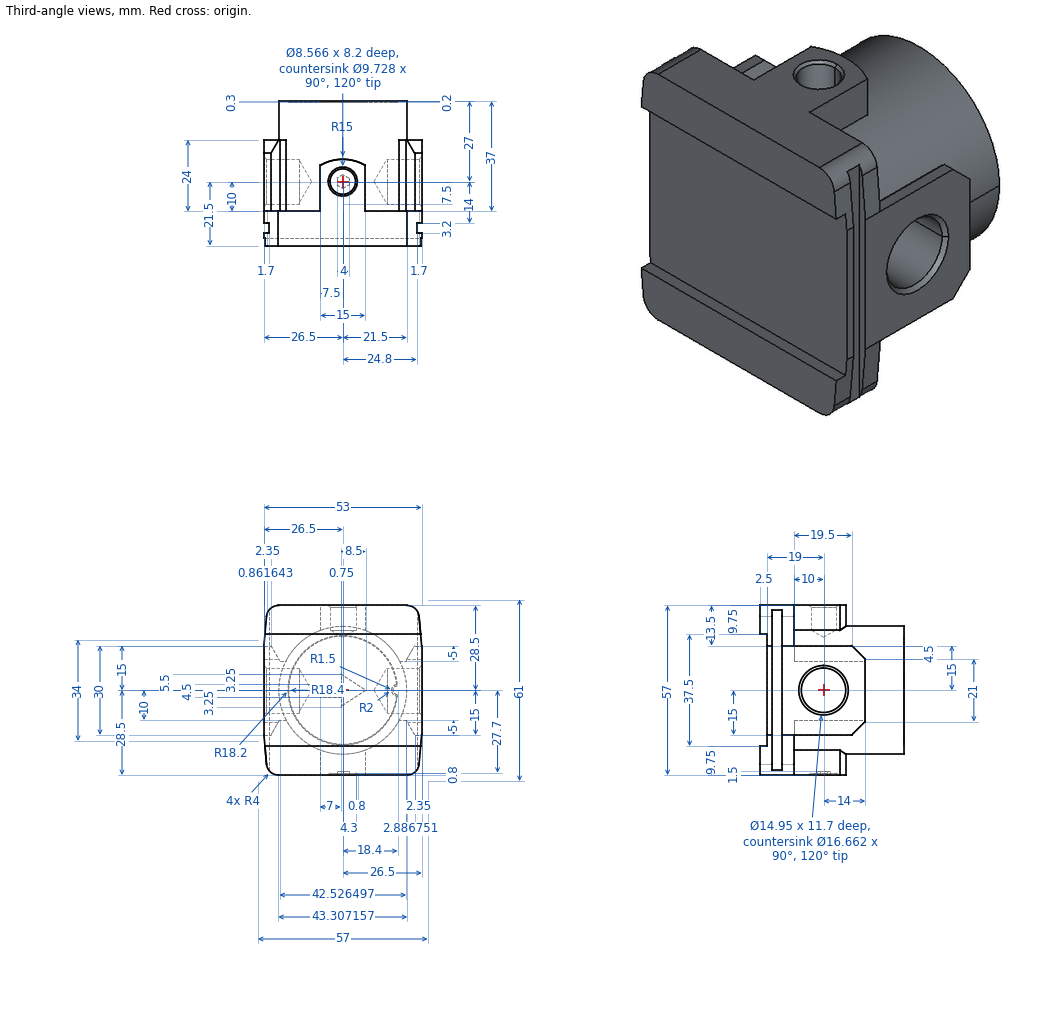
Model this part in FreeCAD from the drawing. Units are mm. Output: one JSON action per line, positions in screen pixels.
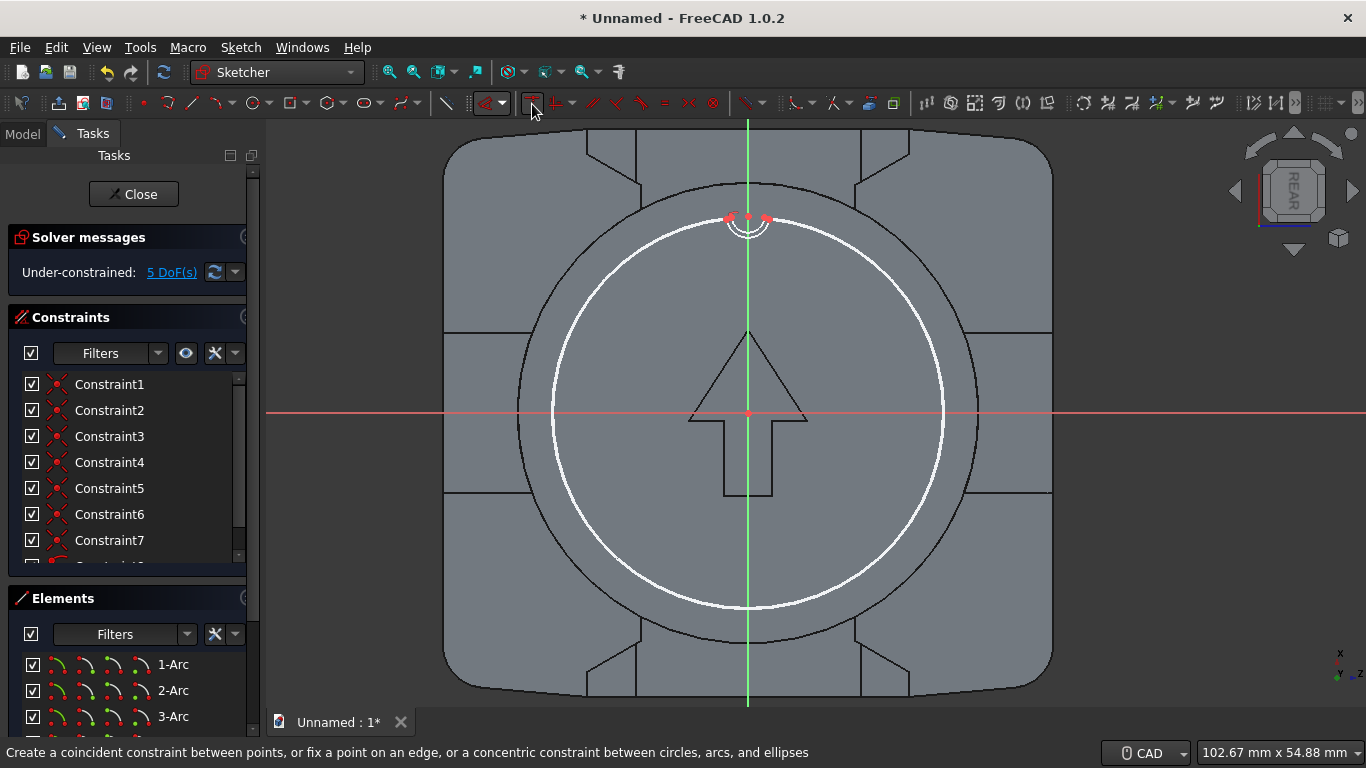
{"action": "scroll", "coordinate": [563, 480], "scroll_direction": "up", "scroll_amount": 12}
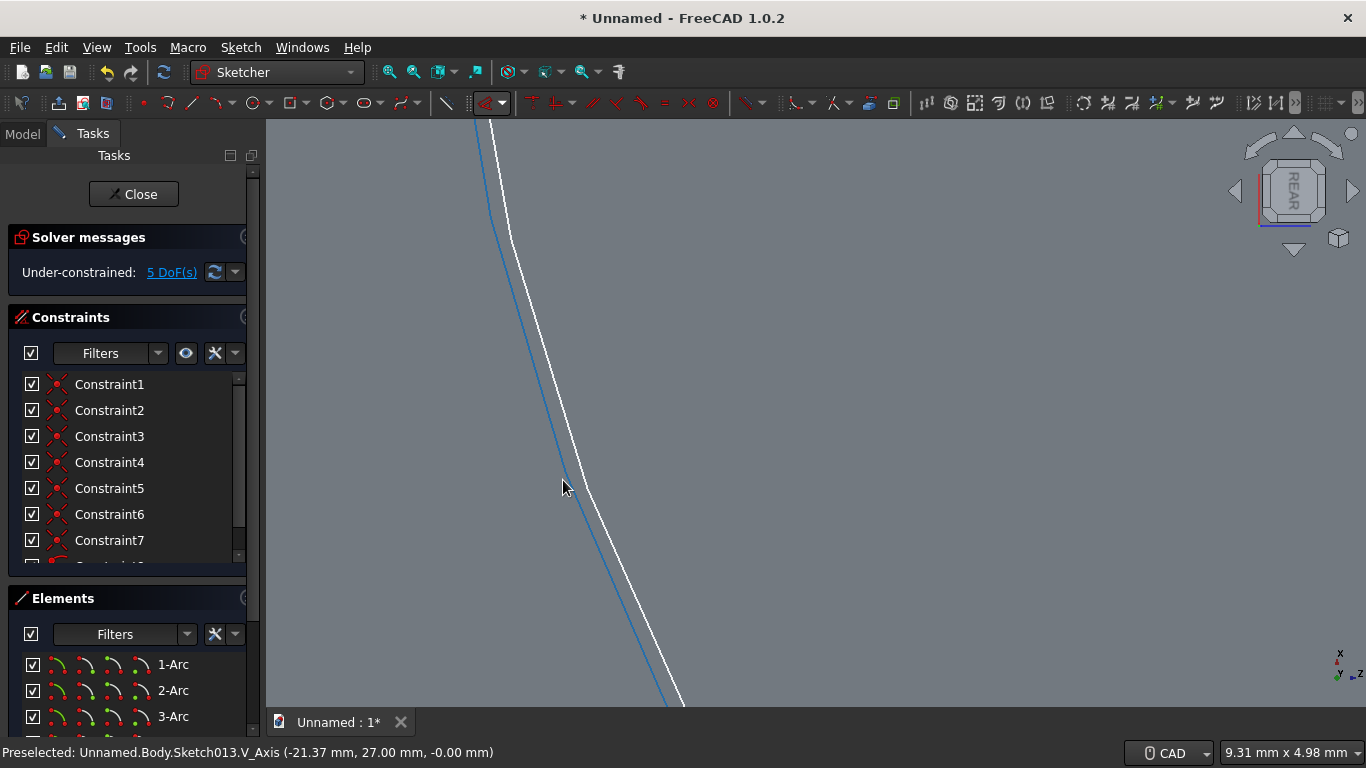
{"action": "left_click", "coordinate": [566, 473]}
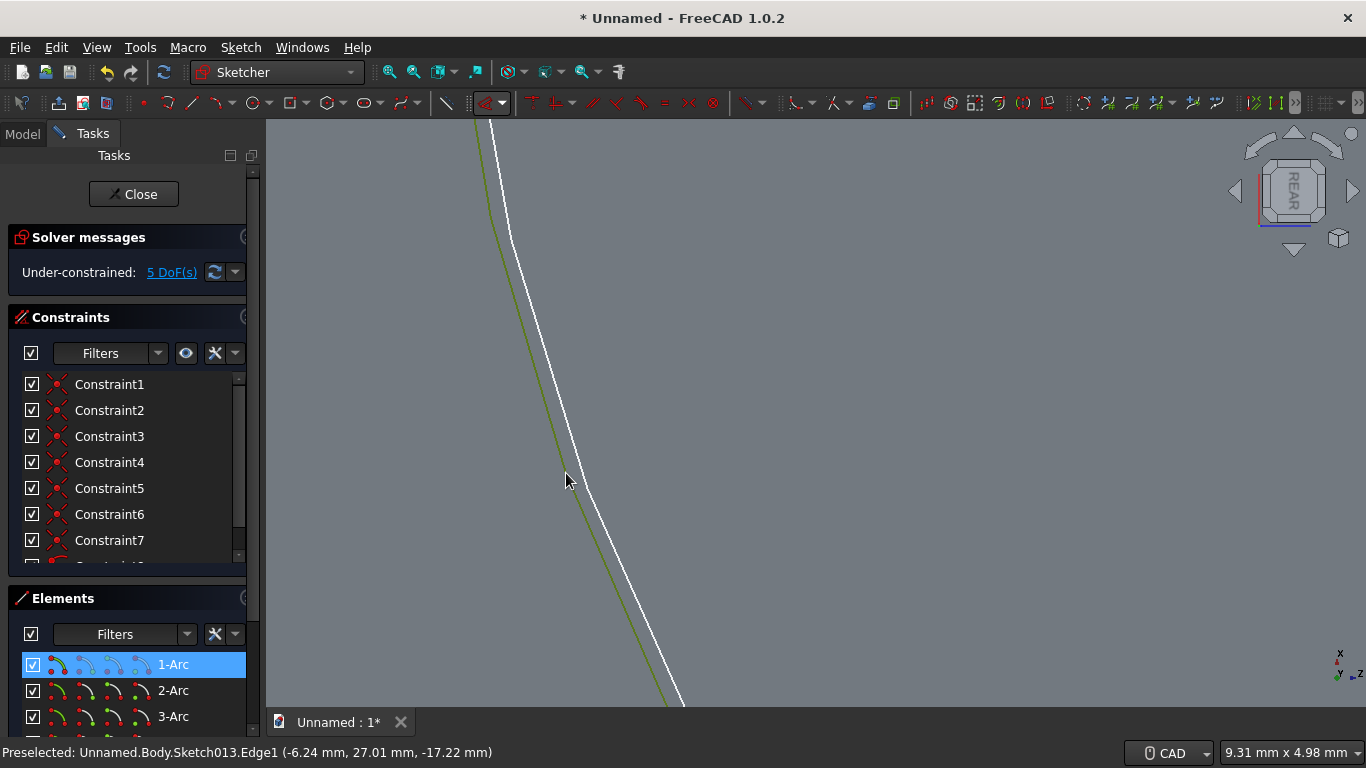
{"action": "left_click", "coordinate": [504, 104]}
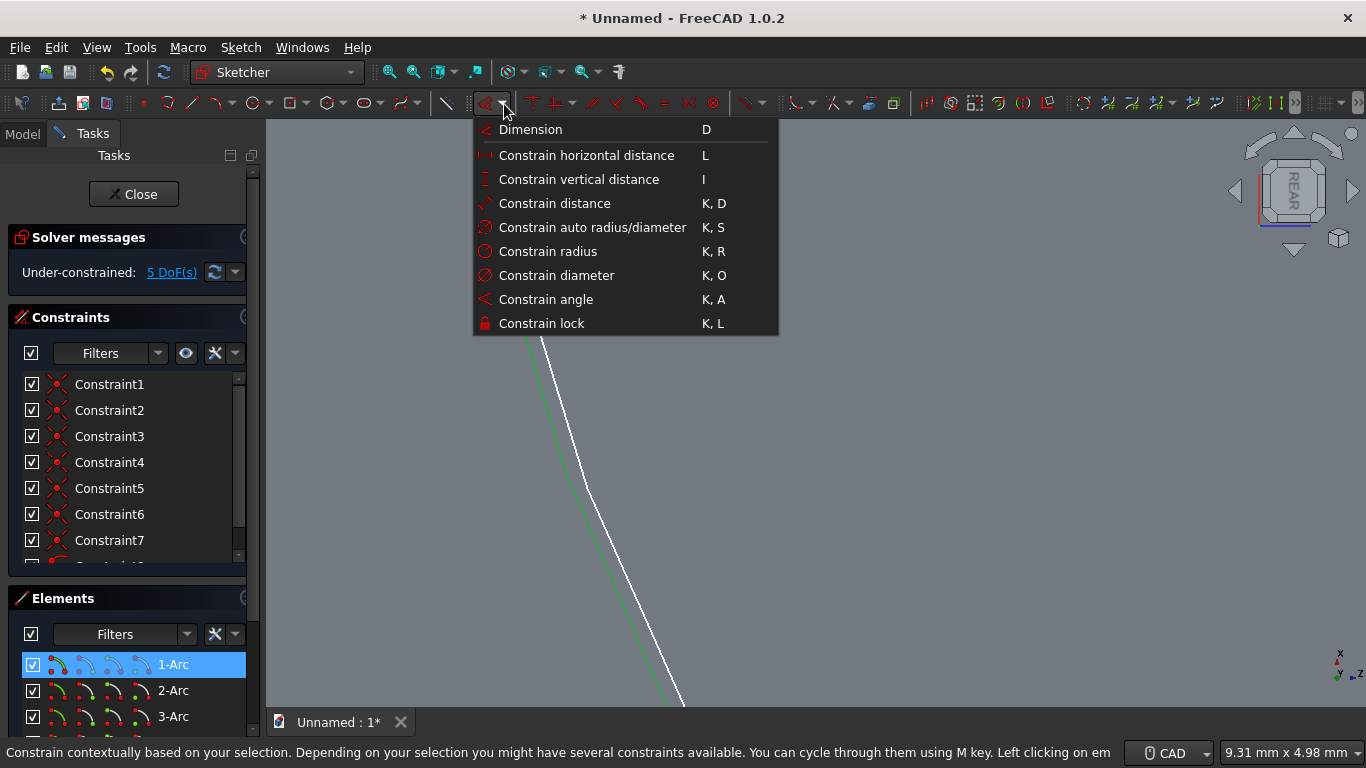
{"action": "left_click", "coordinate": [626, 251]}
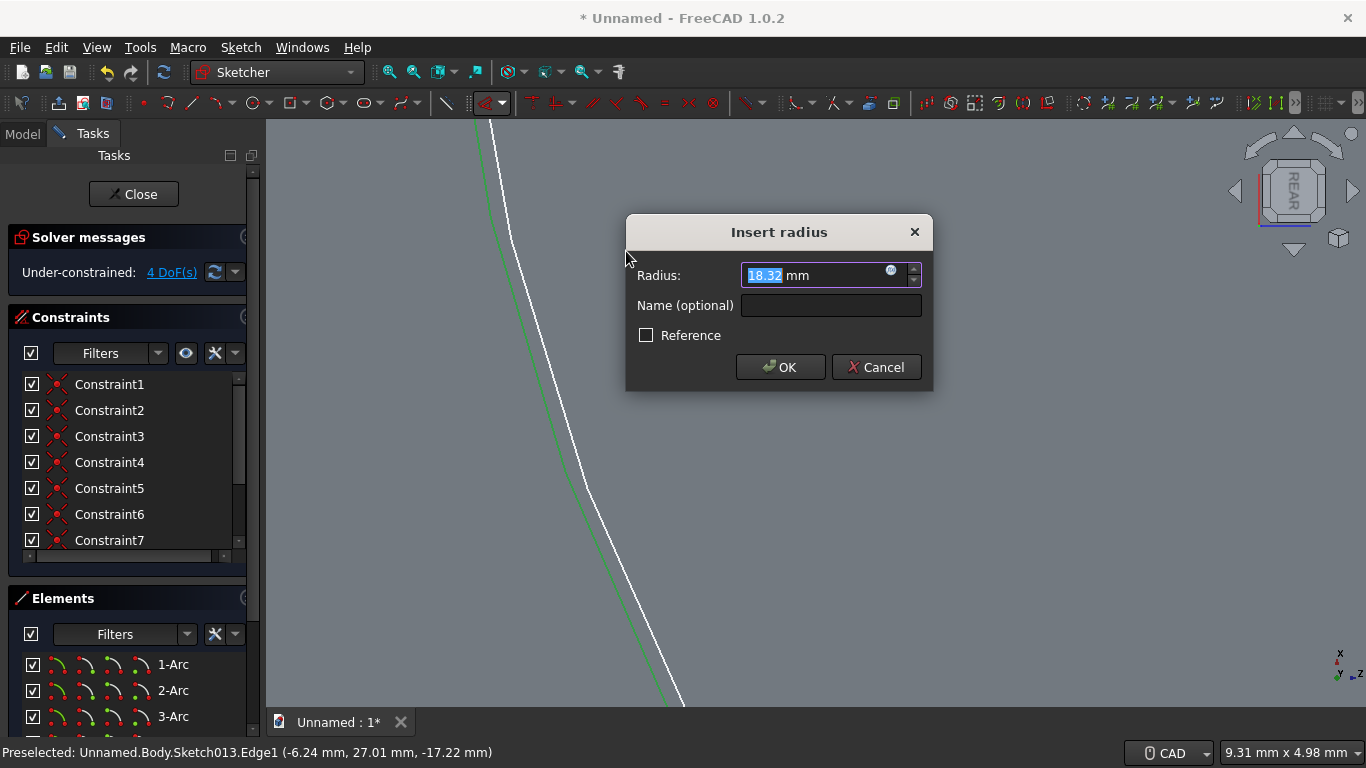
{"action": "type", "text": "18.4"}
{"action": "key", "text": "Return"}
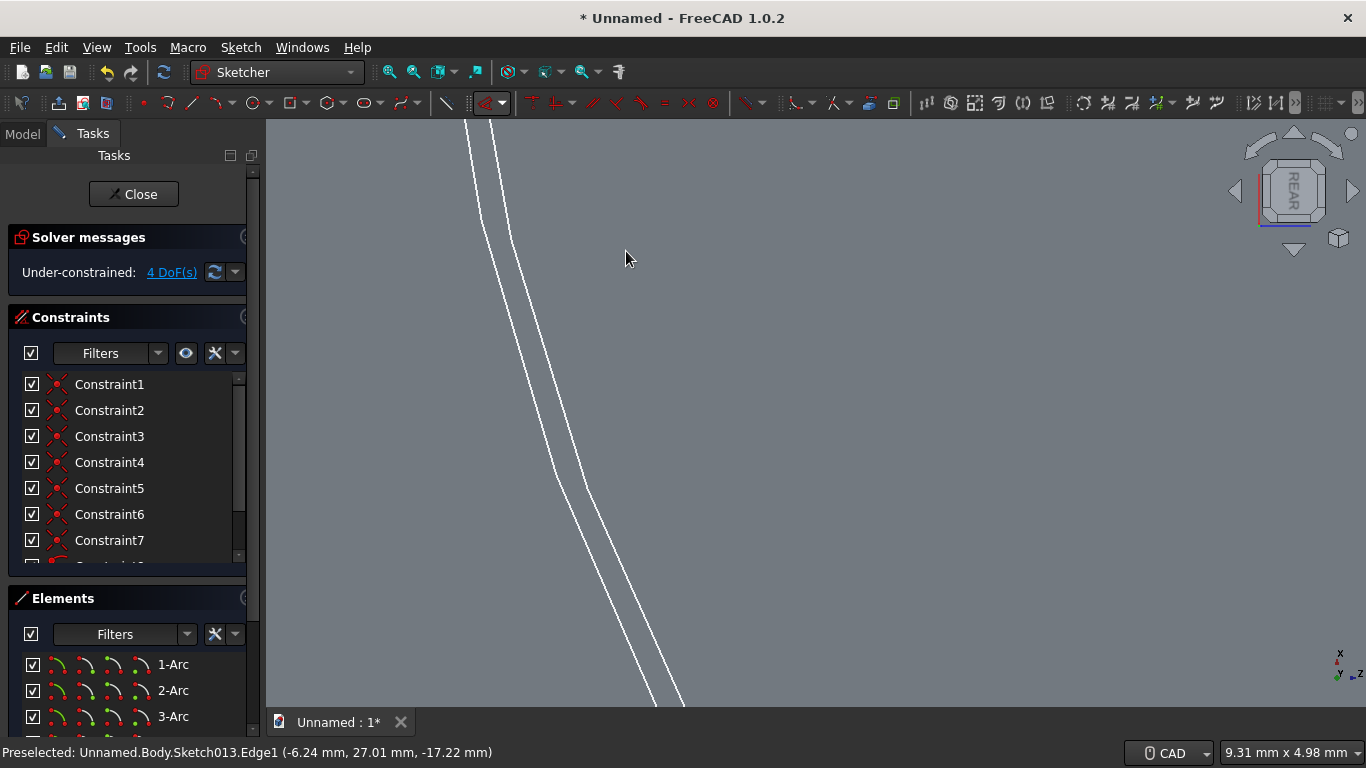
{"action": "scroll", "coordinate": [563, 480], "scroll_direction": "down", "scroll_amount": 12}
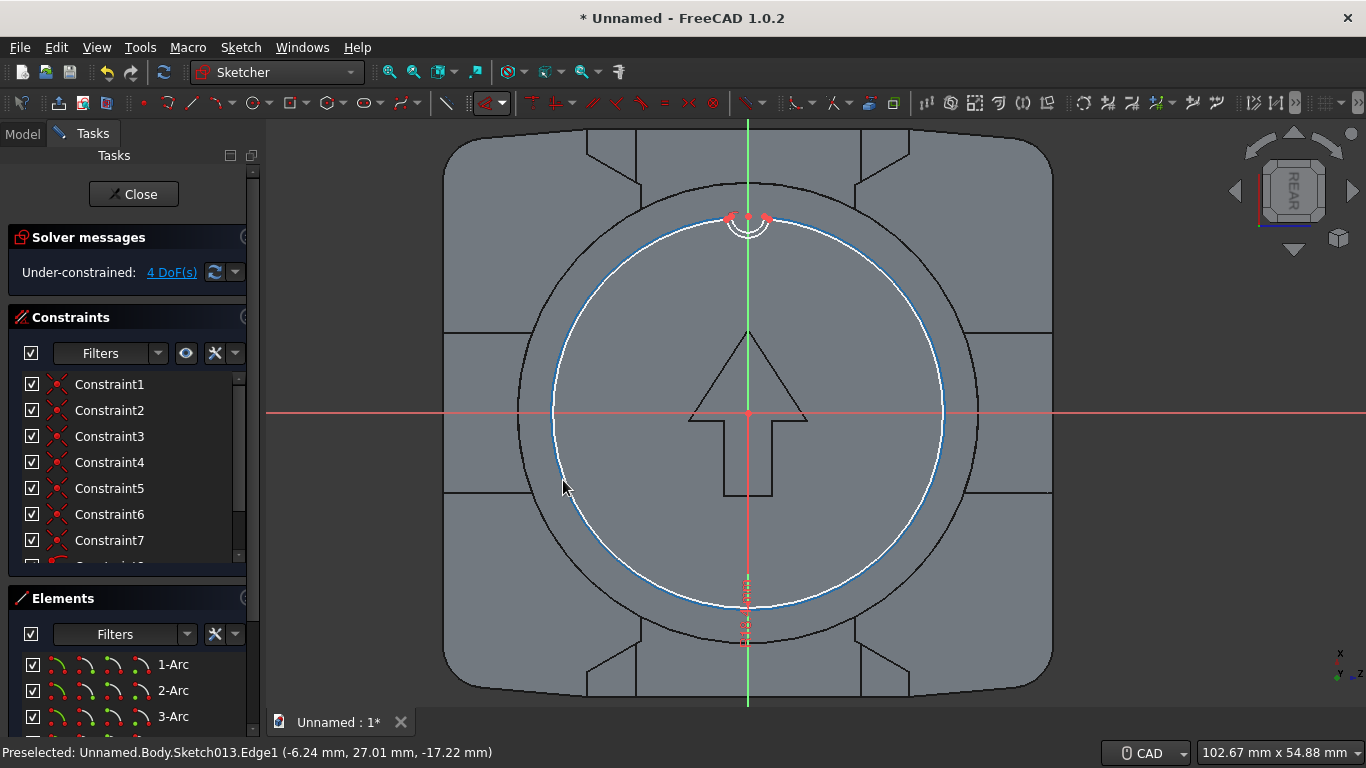
{"action": "scroll", "coordinate": [739, 230], "scroll_direction": "up", "scroll_amount": 5}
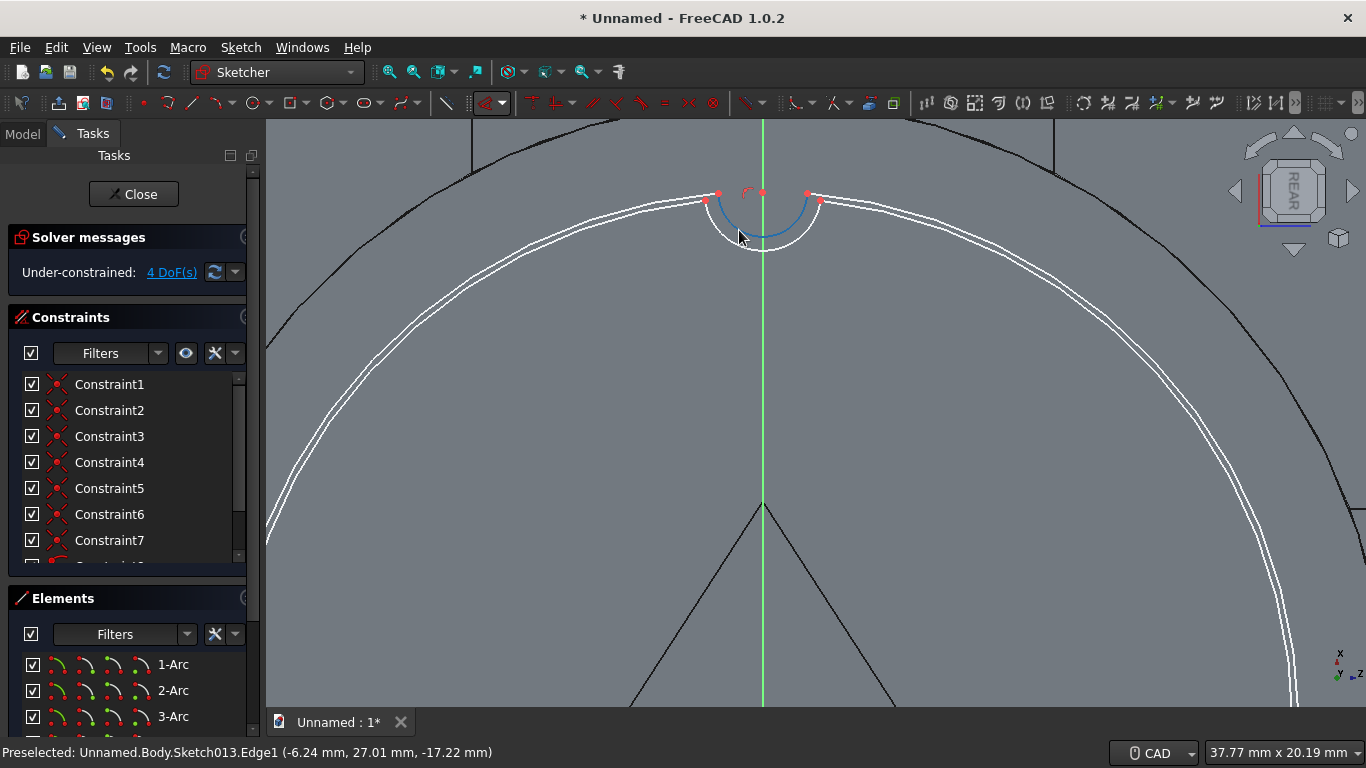
{"action": "left_click", "coordinate": [737, 229]}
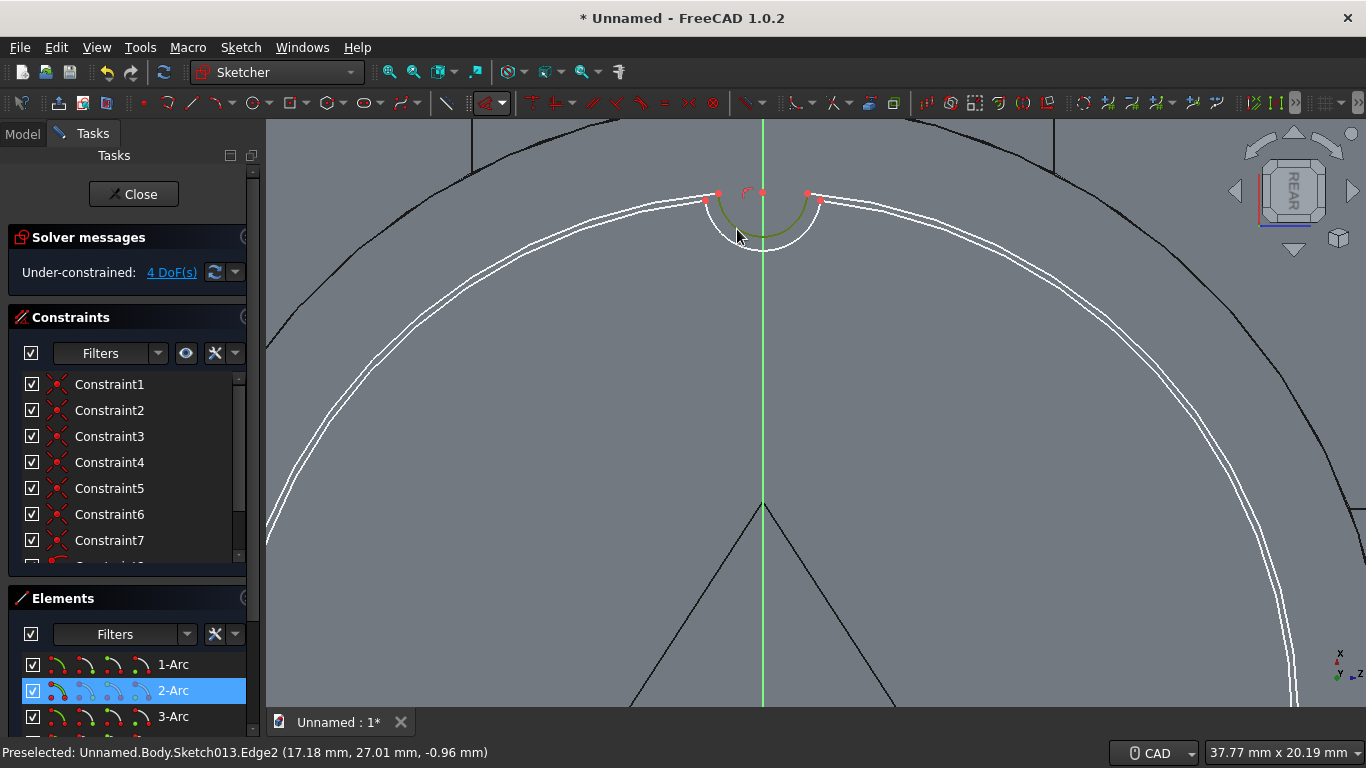
{"action": "left_click", "coordinate": [504, 104]}